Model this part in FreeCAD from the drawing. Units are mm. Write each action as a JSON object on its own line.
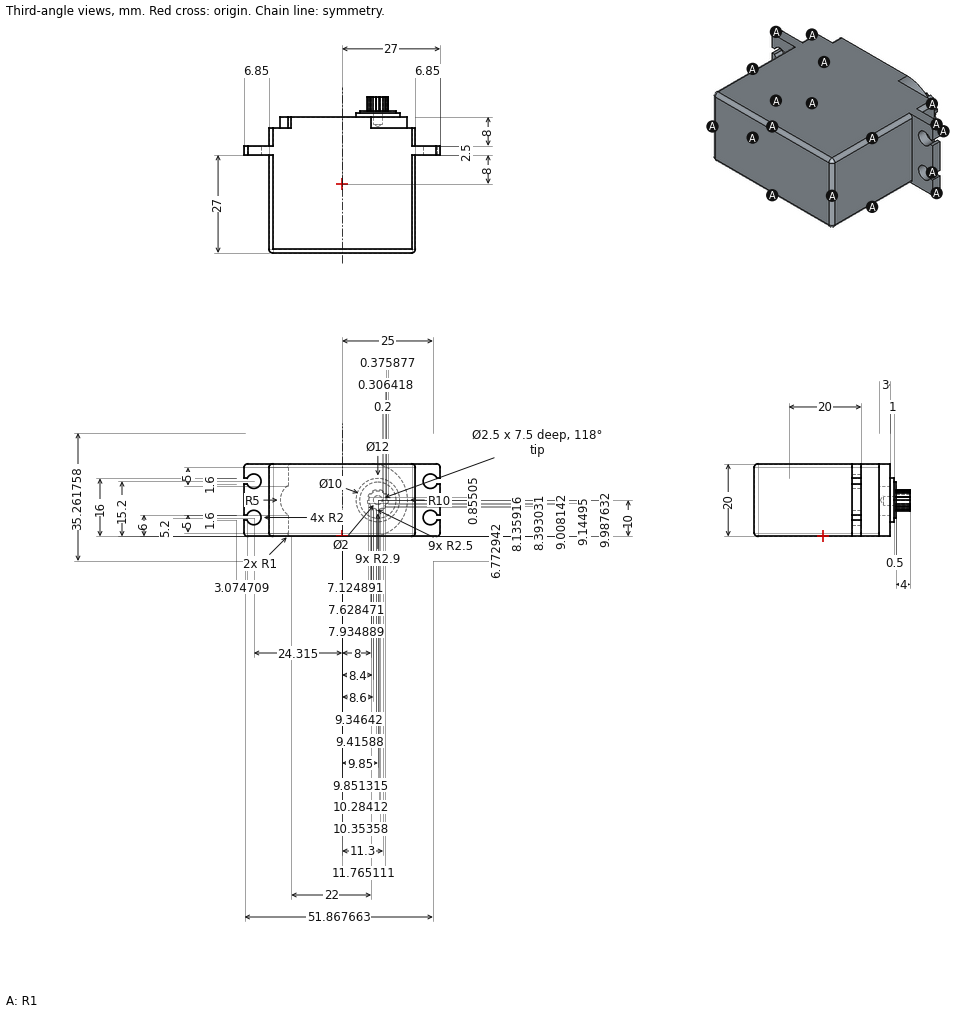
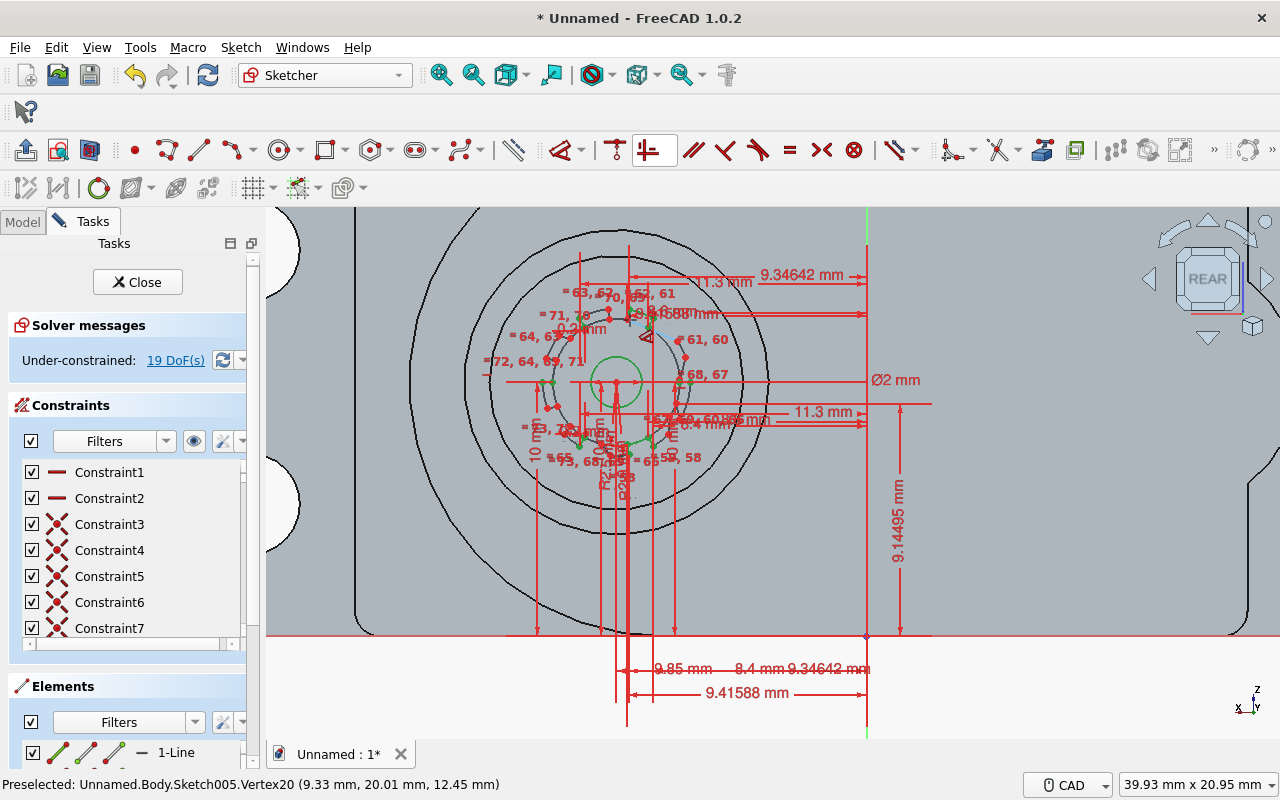
{"action": "left_click", "coordinate": [558, 407]}
{"action": "left_click", "coordinate": [901, 469]}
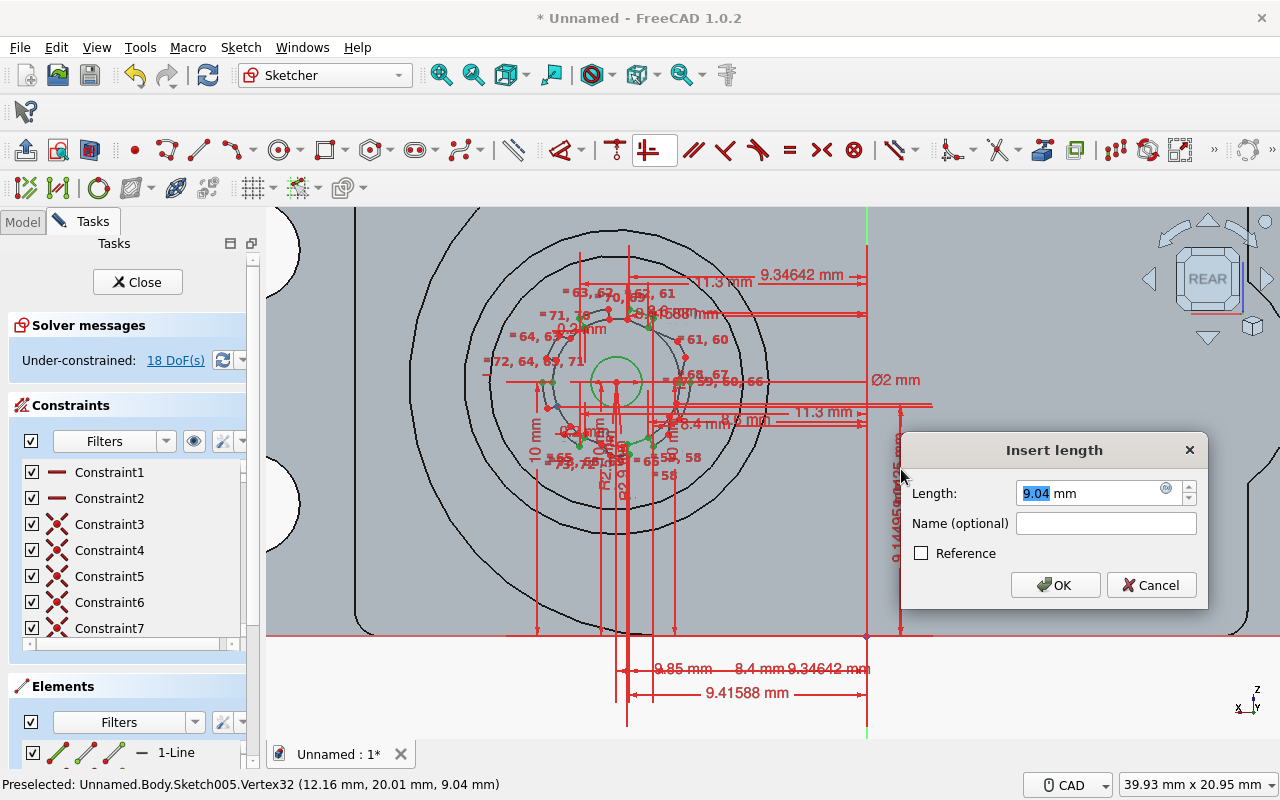
{"action": "type", "text": "9.14495"}
{"action": "key", "text": "Return"}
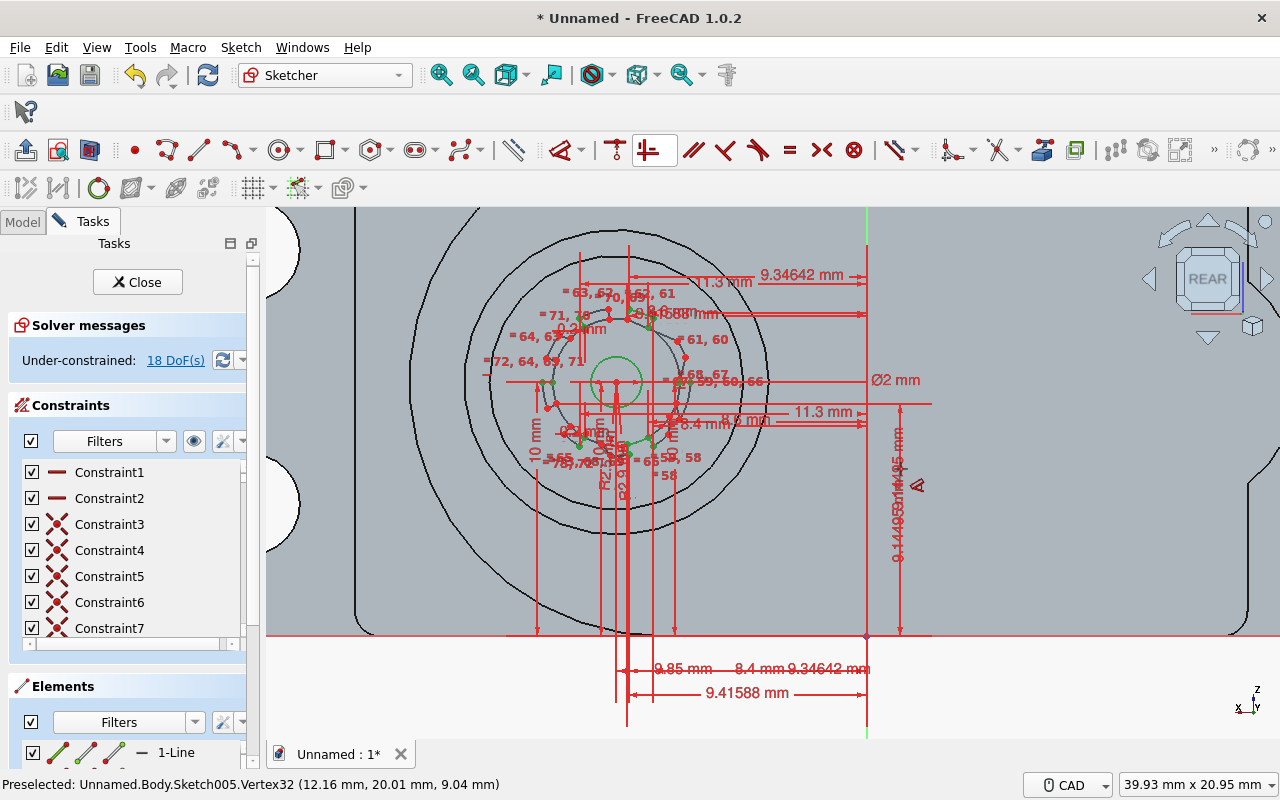
{"action": "scroll", "coordinate": [680, 379], "scroll_direction": "up", "scroll_amount": 8}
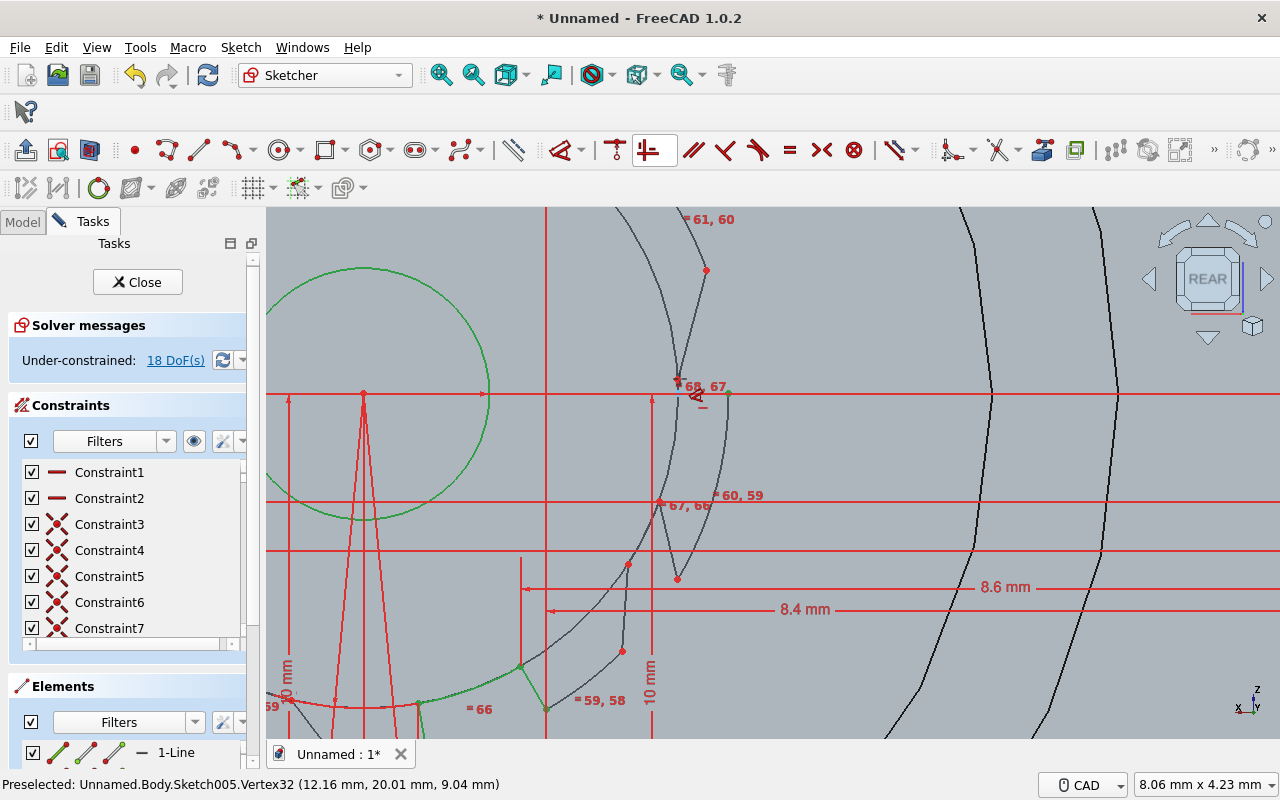
{"action": "left_click", "coordinate": [678, 380]}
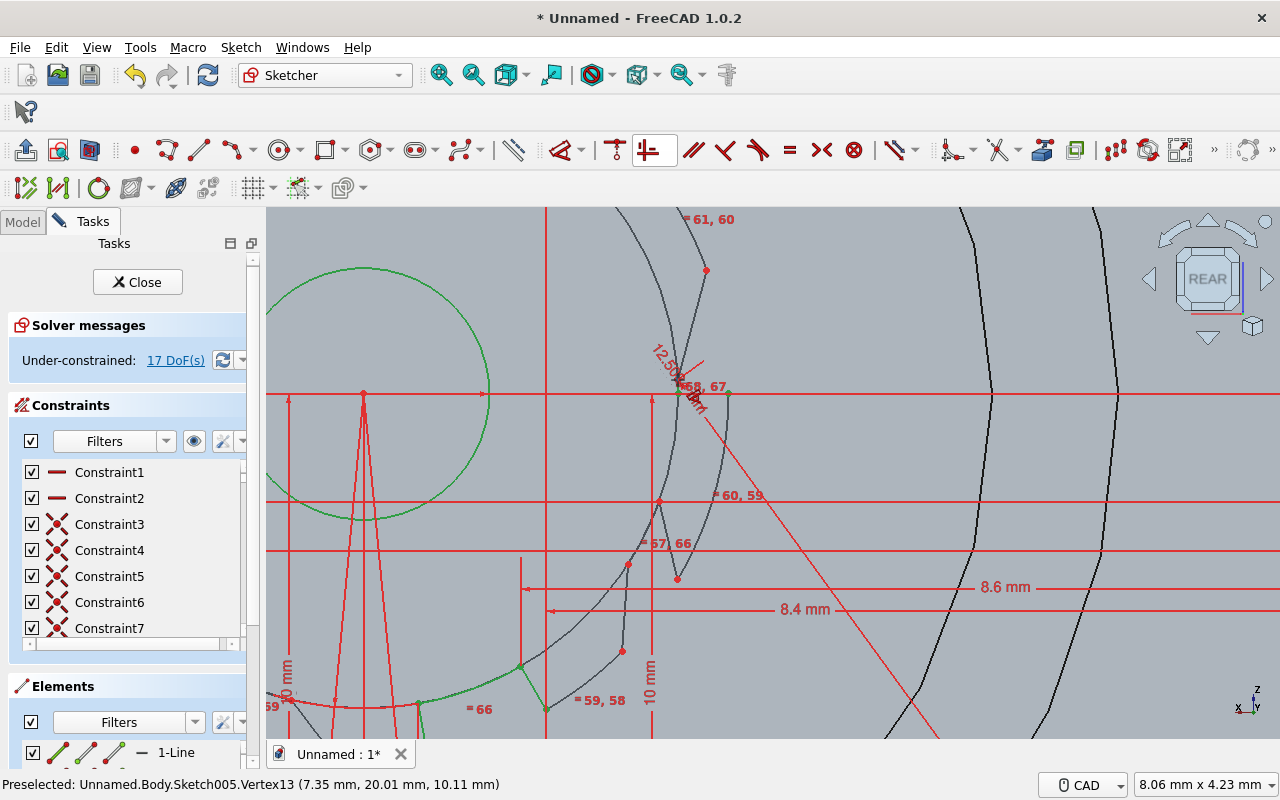
{"action": "left_click", "coordinate": [364, 394]}
{"action": "left_click", "coordinate": [330, 387]}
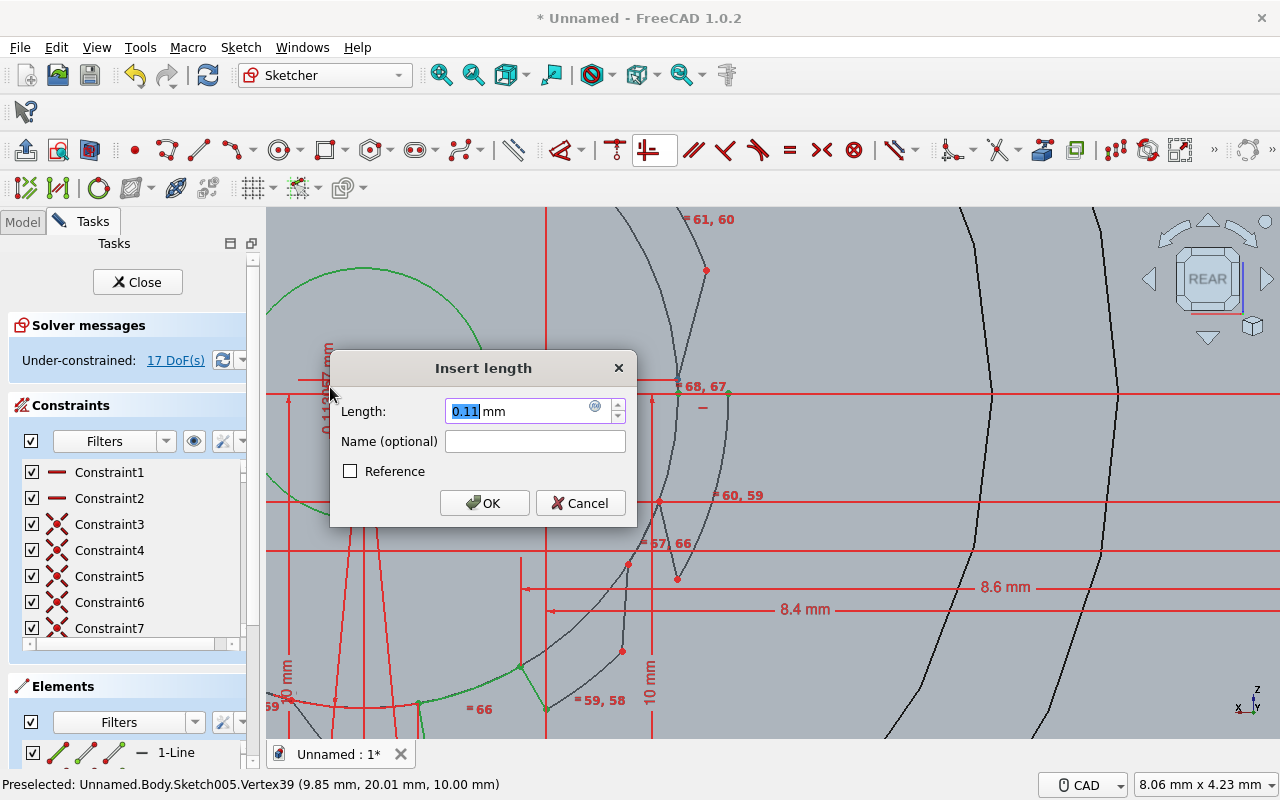
{"action": "type", "text": "0.85505"}
{"action": "key", "text": "Return"}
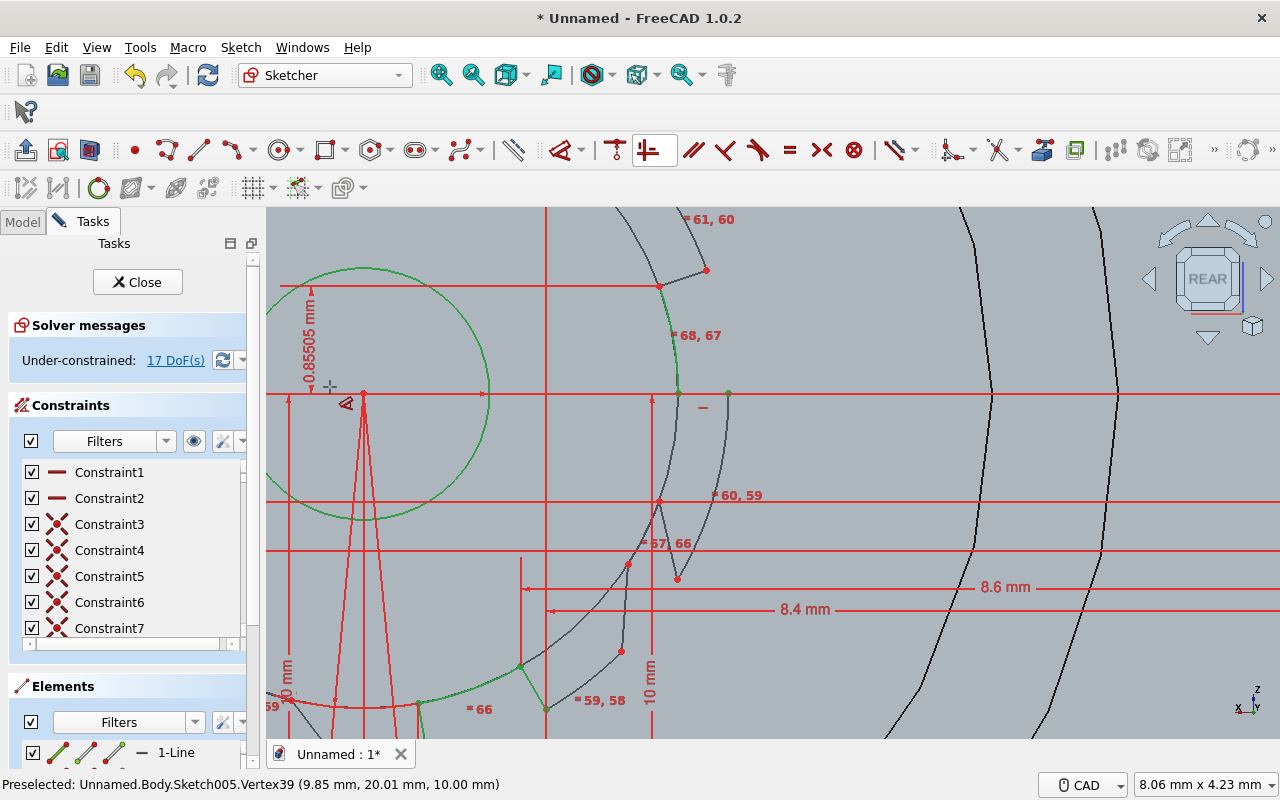
{"action": "scroll", "coordinate": [680, 379], "scroll_direction": "down", "scroll_amount": 8}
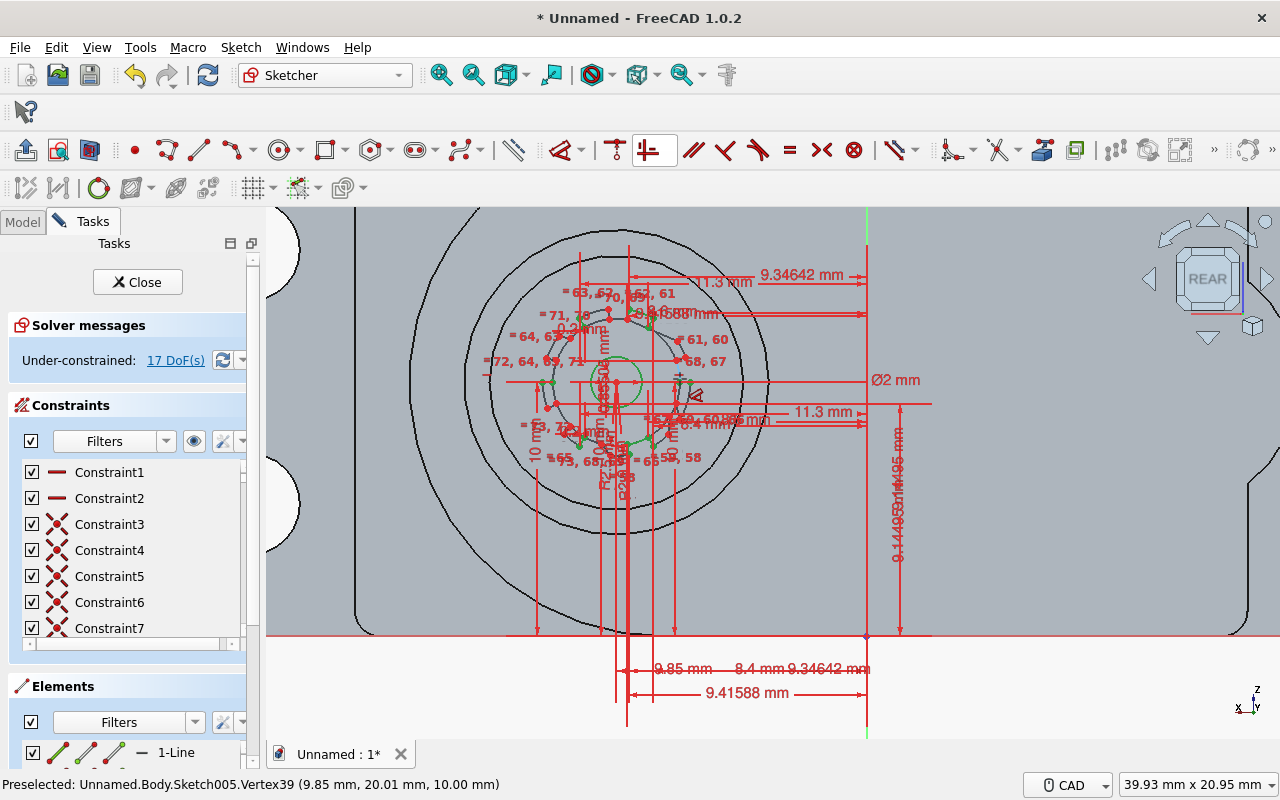
{"action": "scroll", "coordinate": [557, 361], "scroll_direction": "up", "scroll_amount": 4}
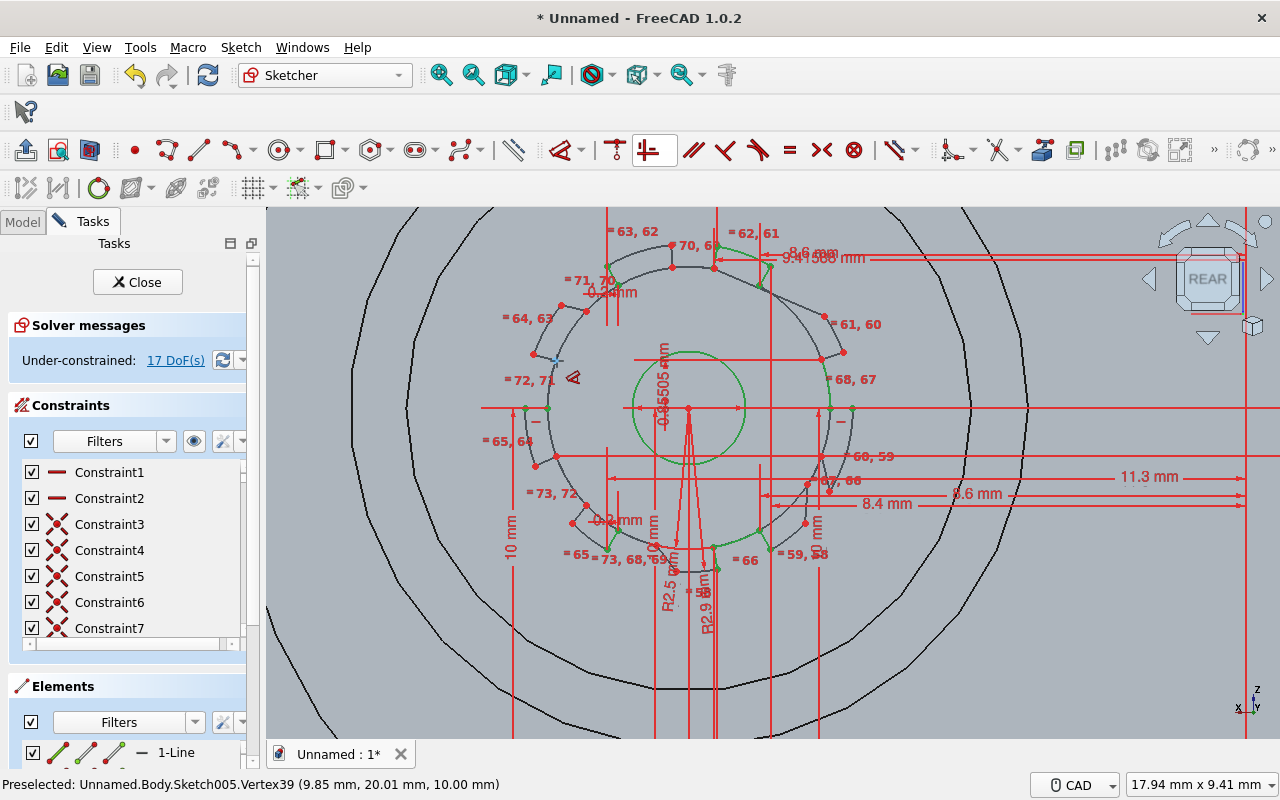
{"action": "left_click", "coordinate": [556, 360]}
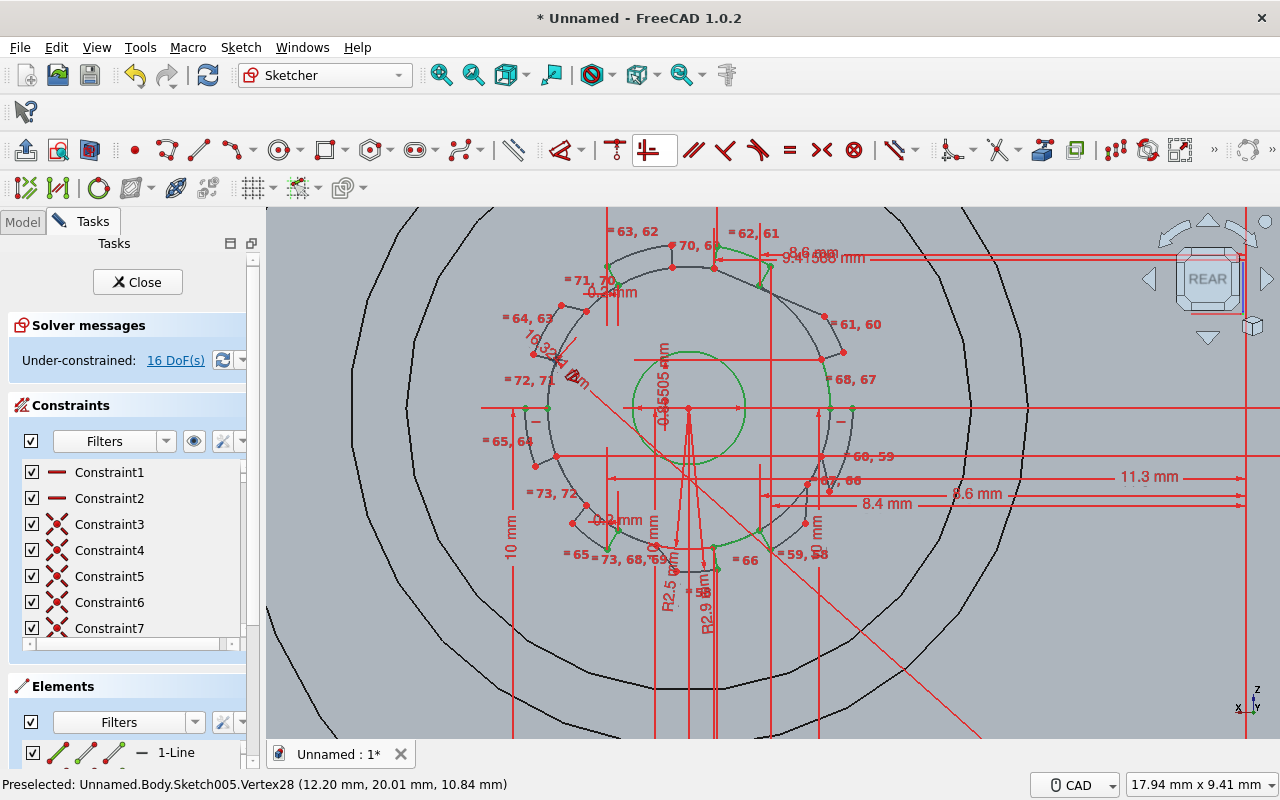
{"action": "left_click", "coordinate": [689, 408]}
{"action": "left_click", "coordinate": [522, 384]}